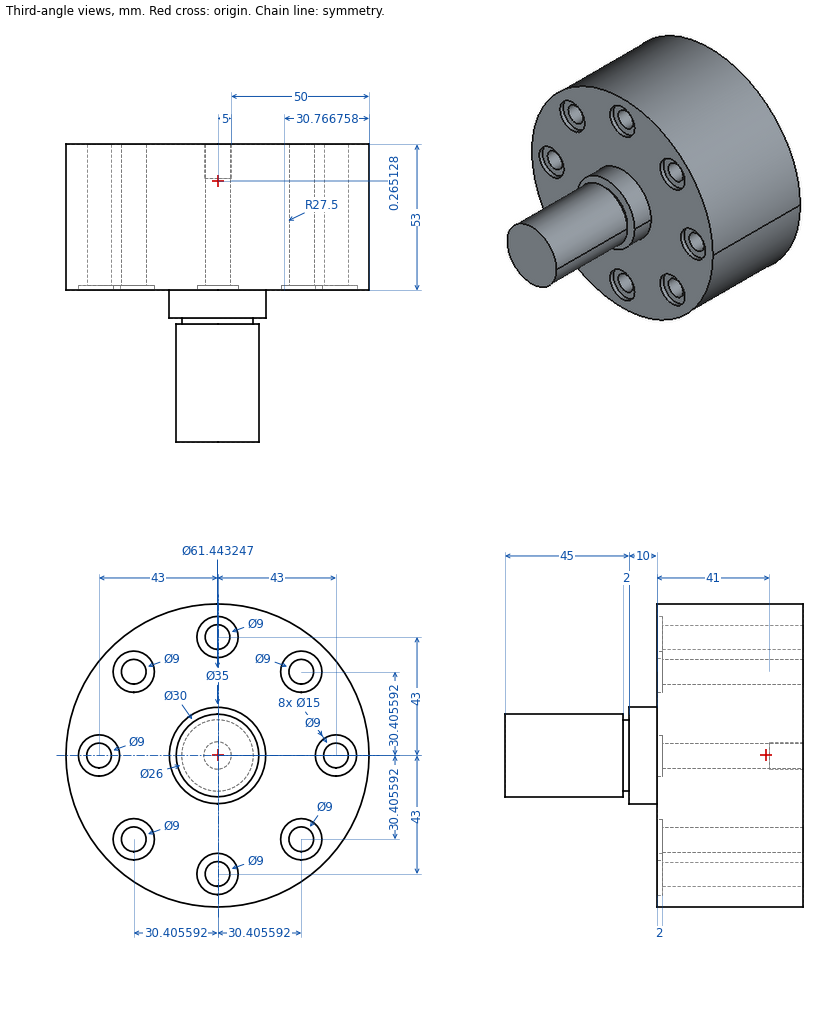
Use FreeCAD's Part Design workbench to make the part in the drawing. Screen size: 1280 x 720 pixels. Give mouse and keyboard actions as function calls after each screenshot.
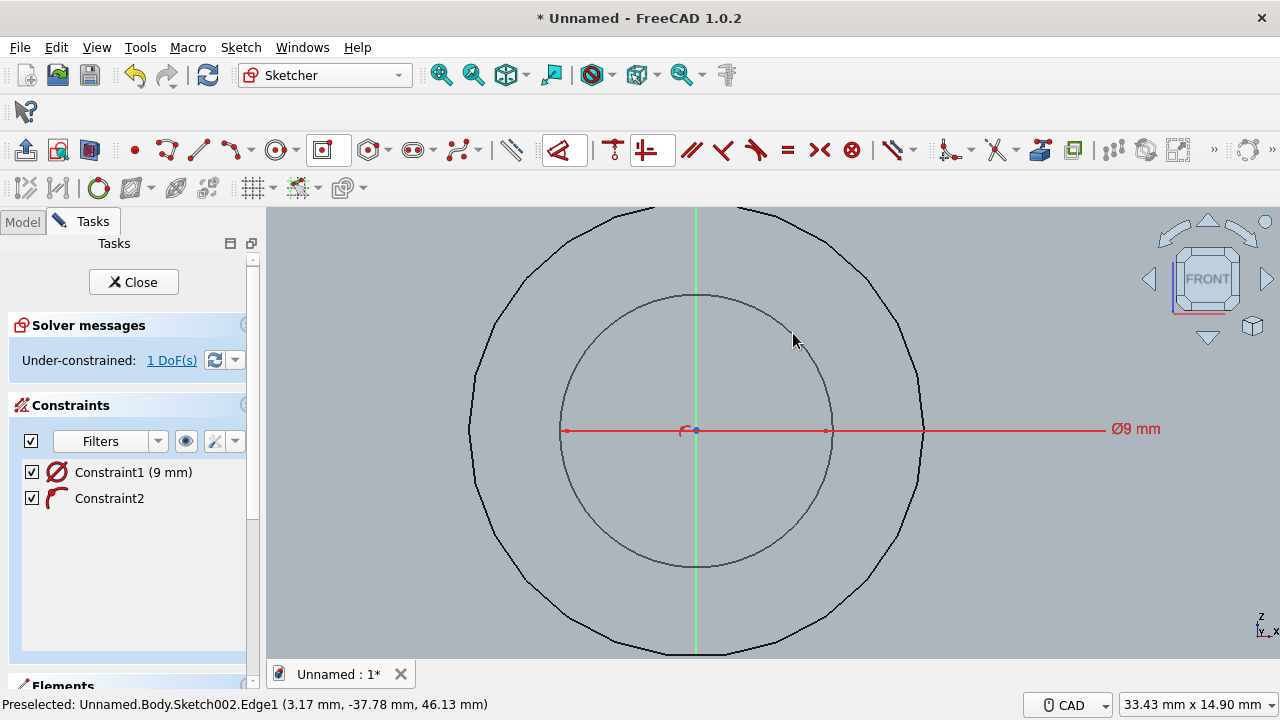
click(696, 431)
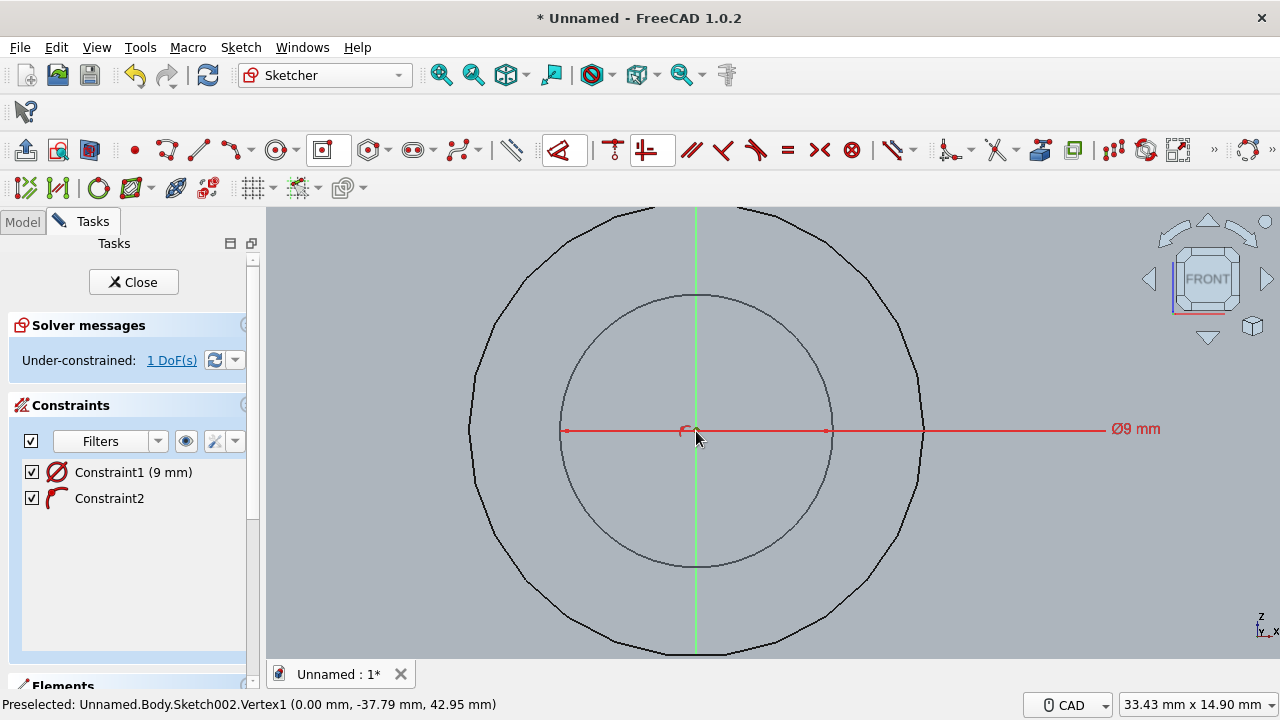
key(i)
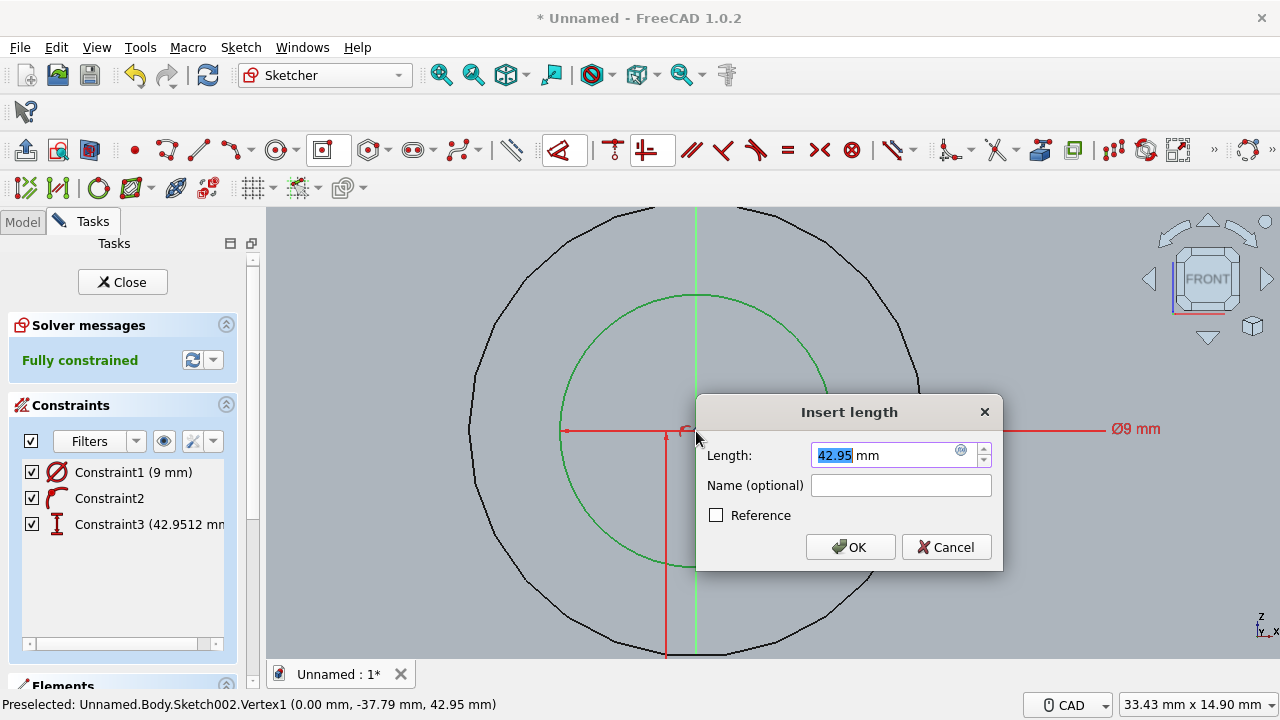
text(43)
key(Return)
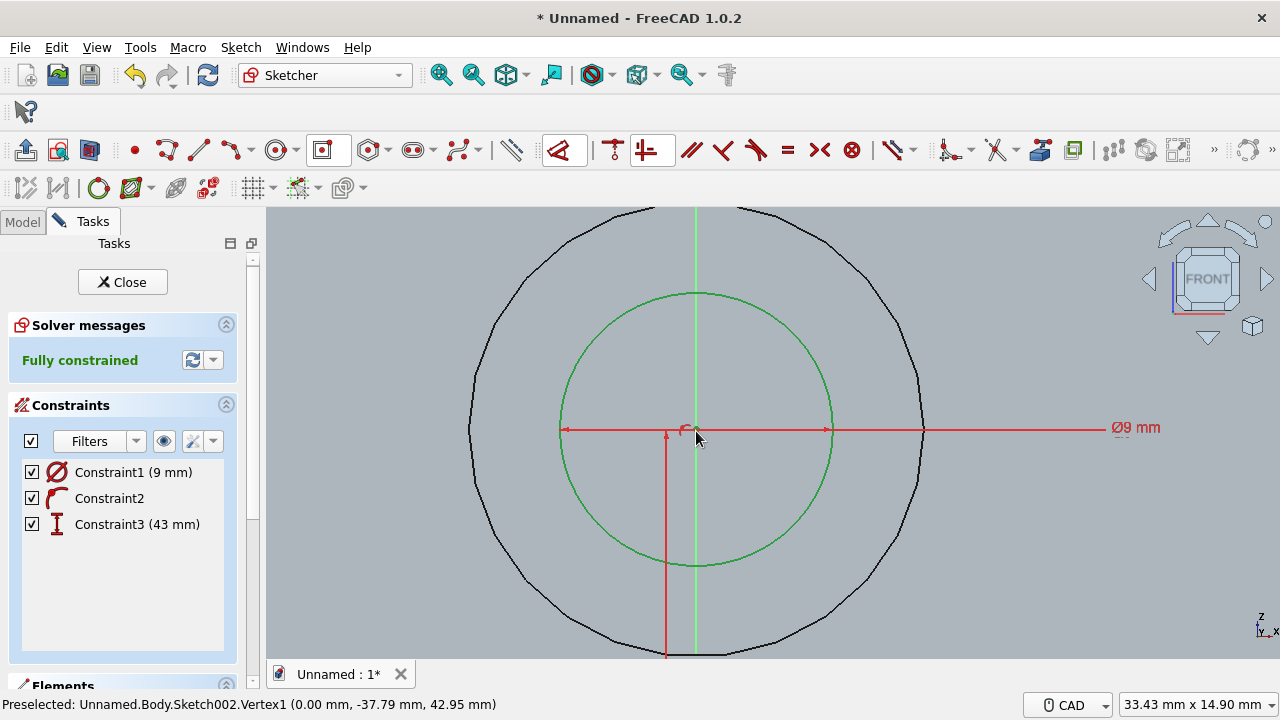
click(123, 282)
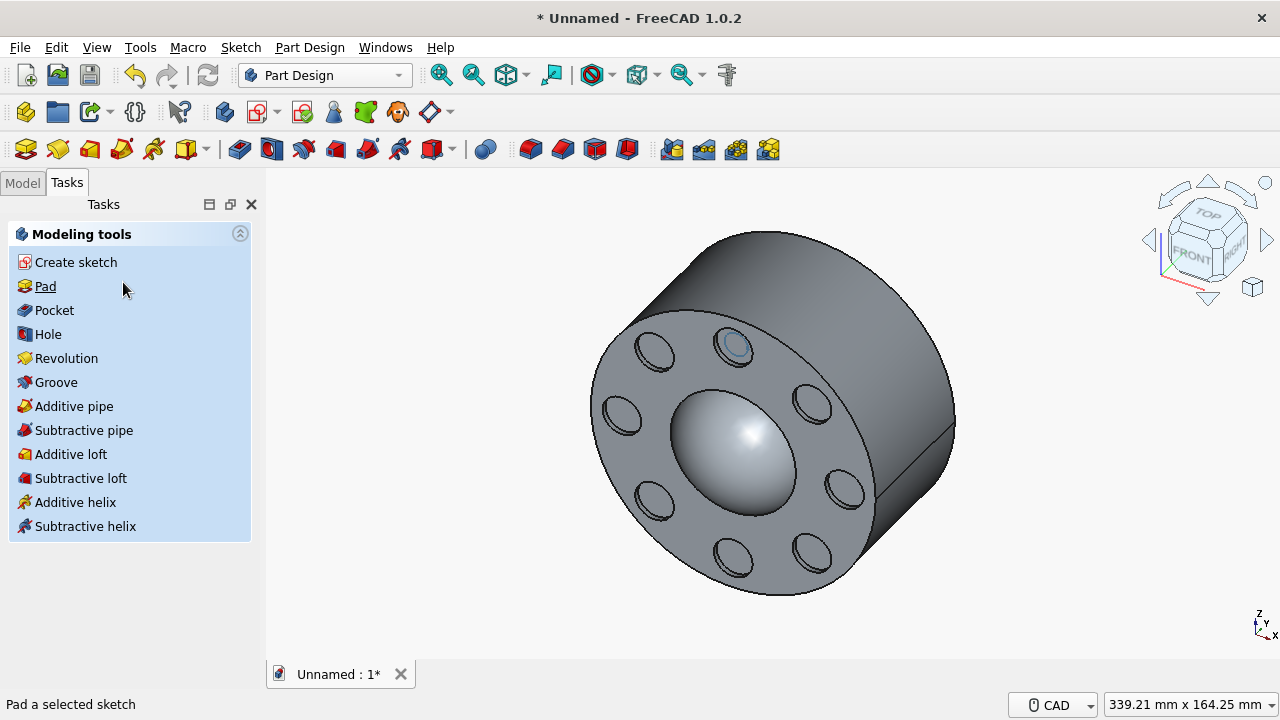
click(240, 150)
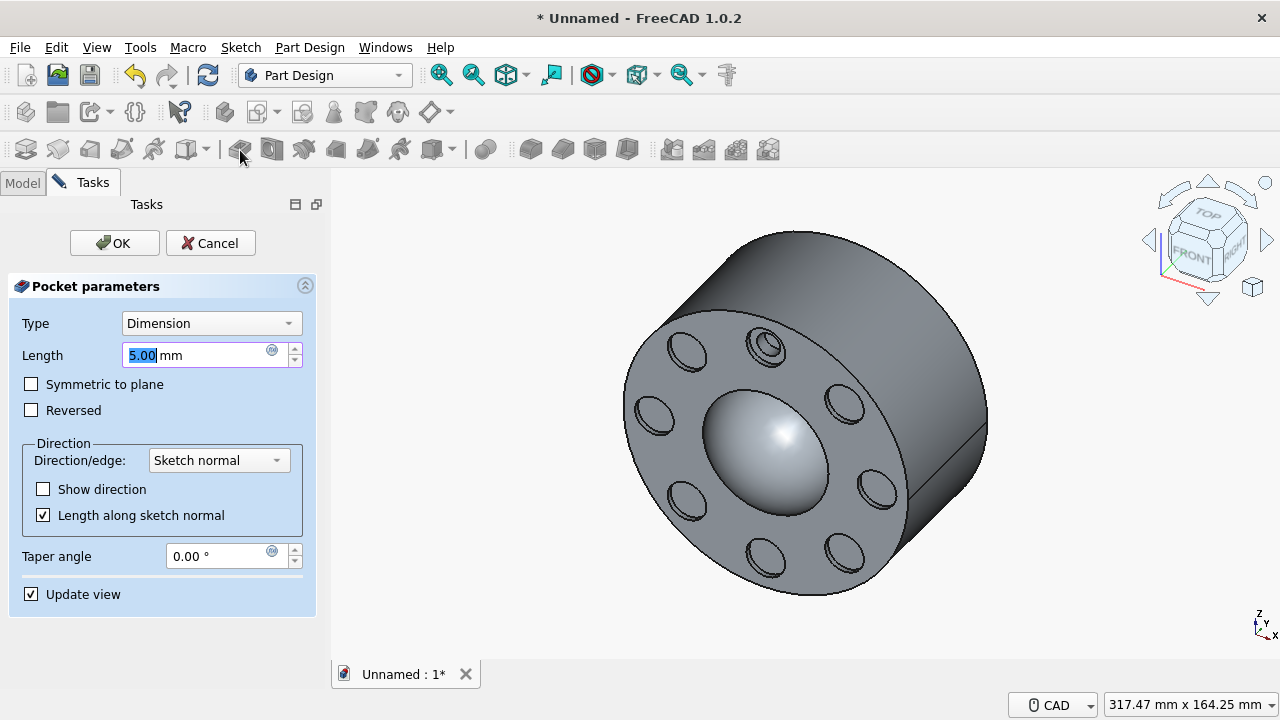
click(212, 324)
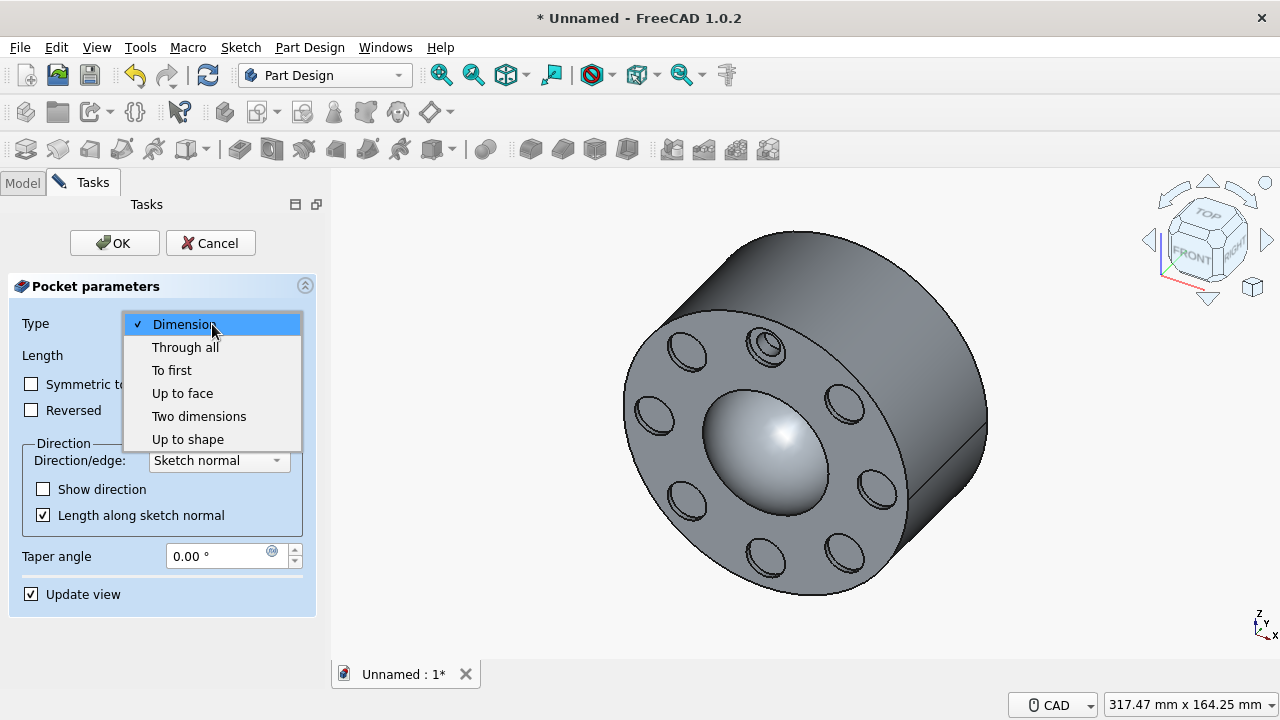
click(212, 370)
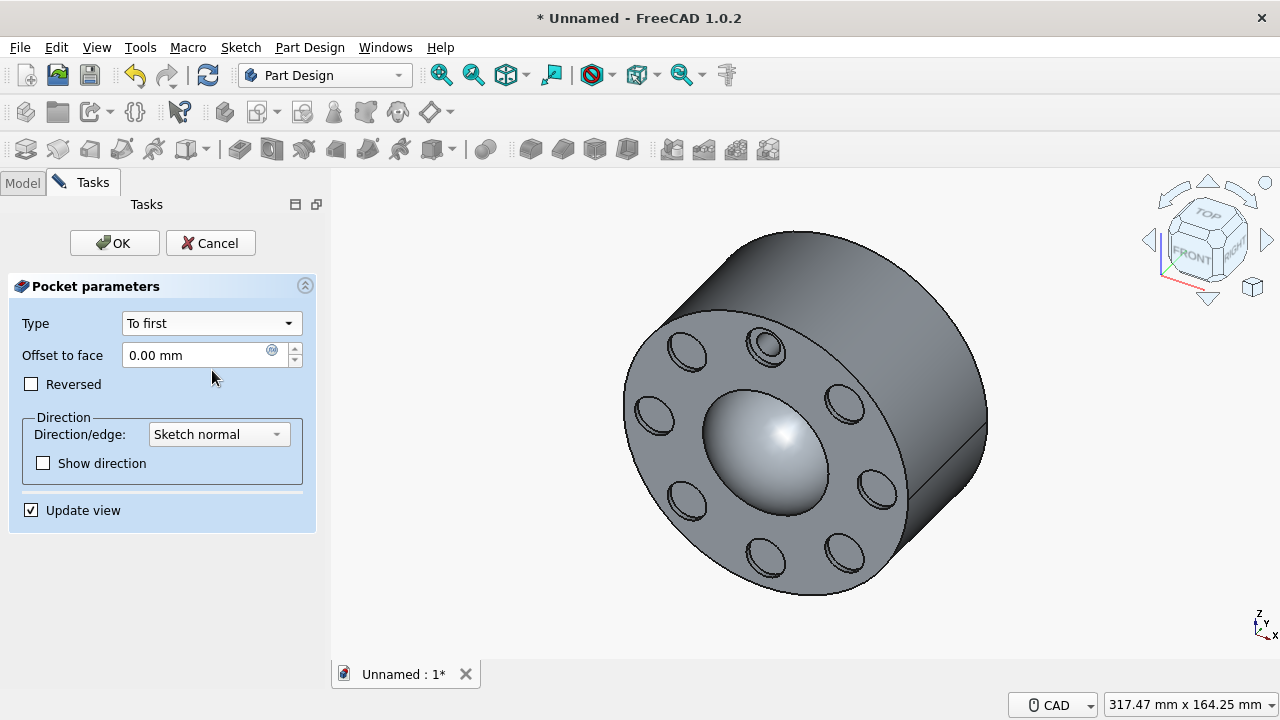
click(115, 243)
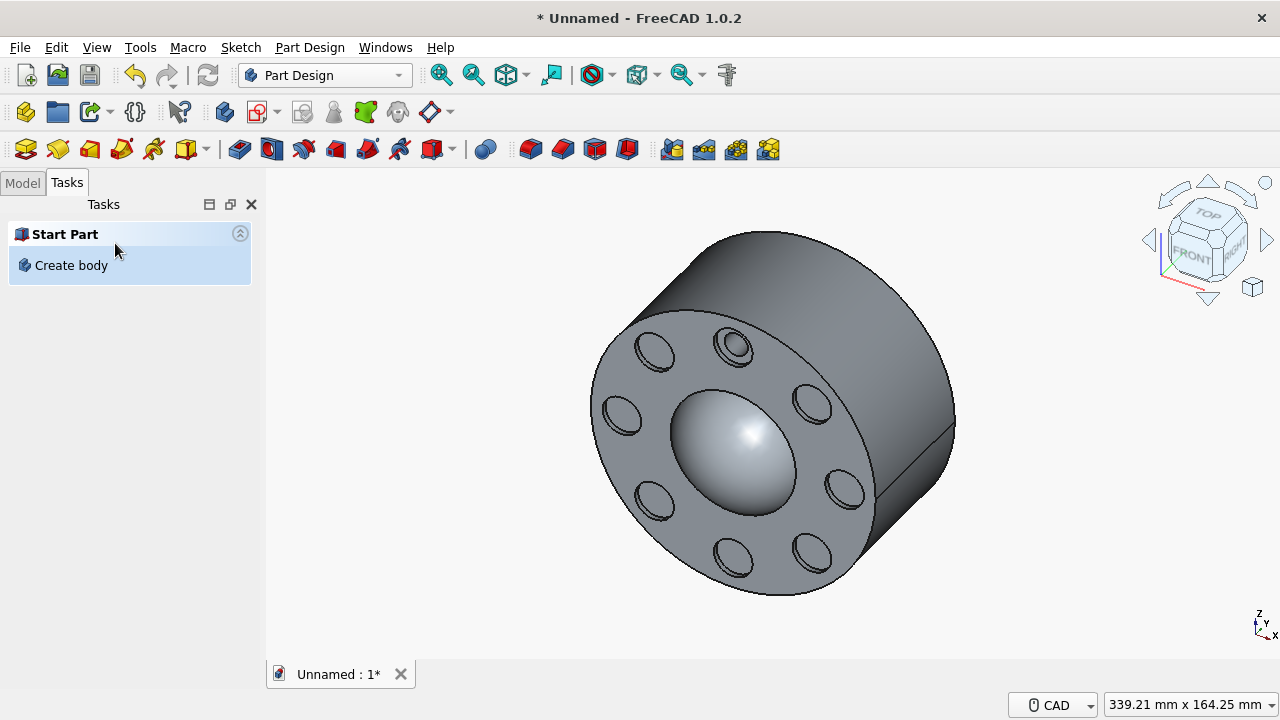
click(658, 348)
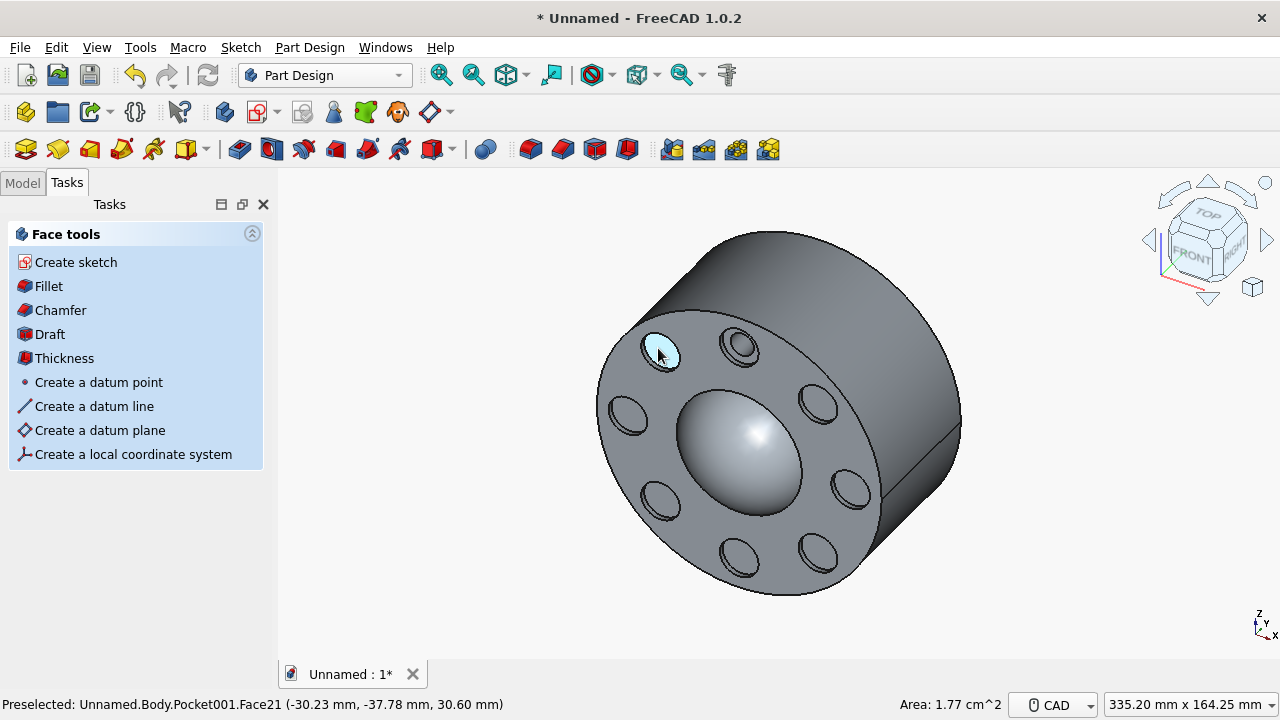
click(258, 112)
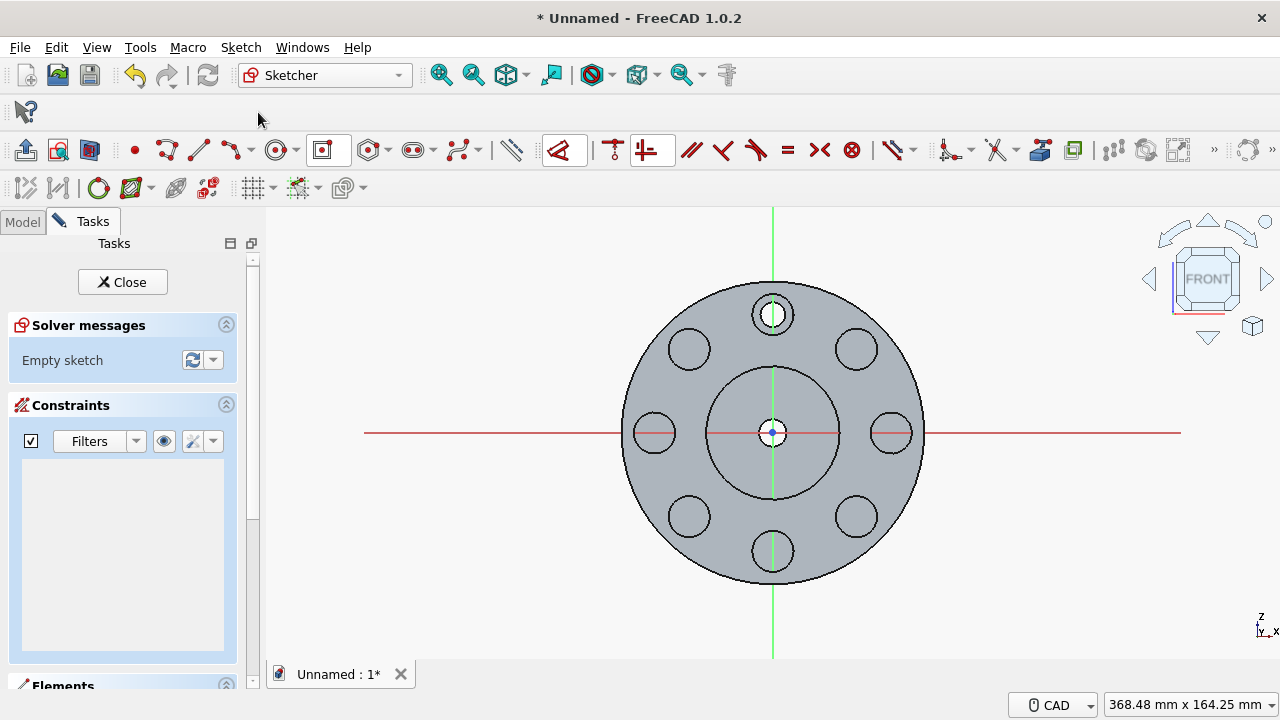
scroll(872, 341, up, 12)